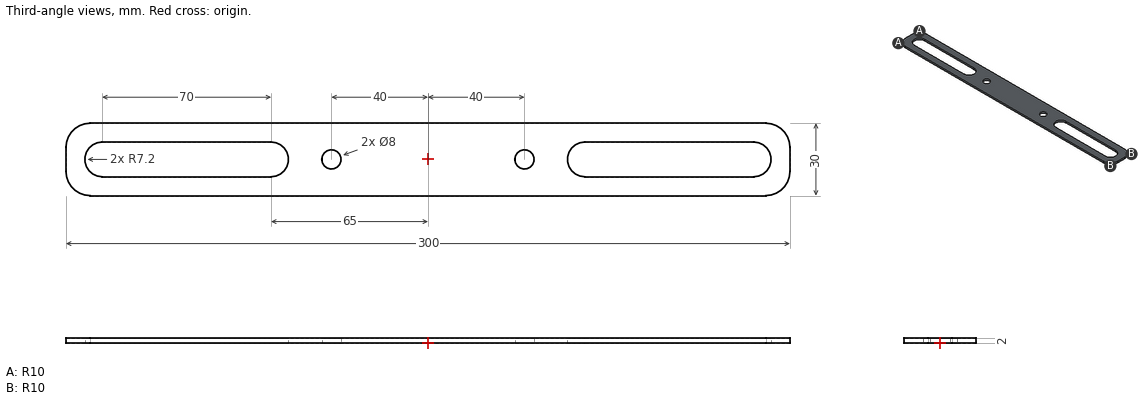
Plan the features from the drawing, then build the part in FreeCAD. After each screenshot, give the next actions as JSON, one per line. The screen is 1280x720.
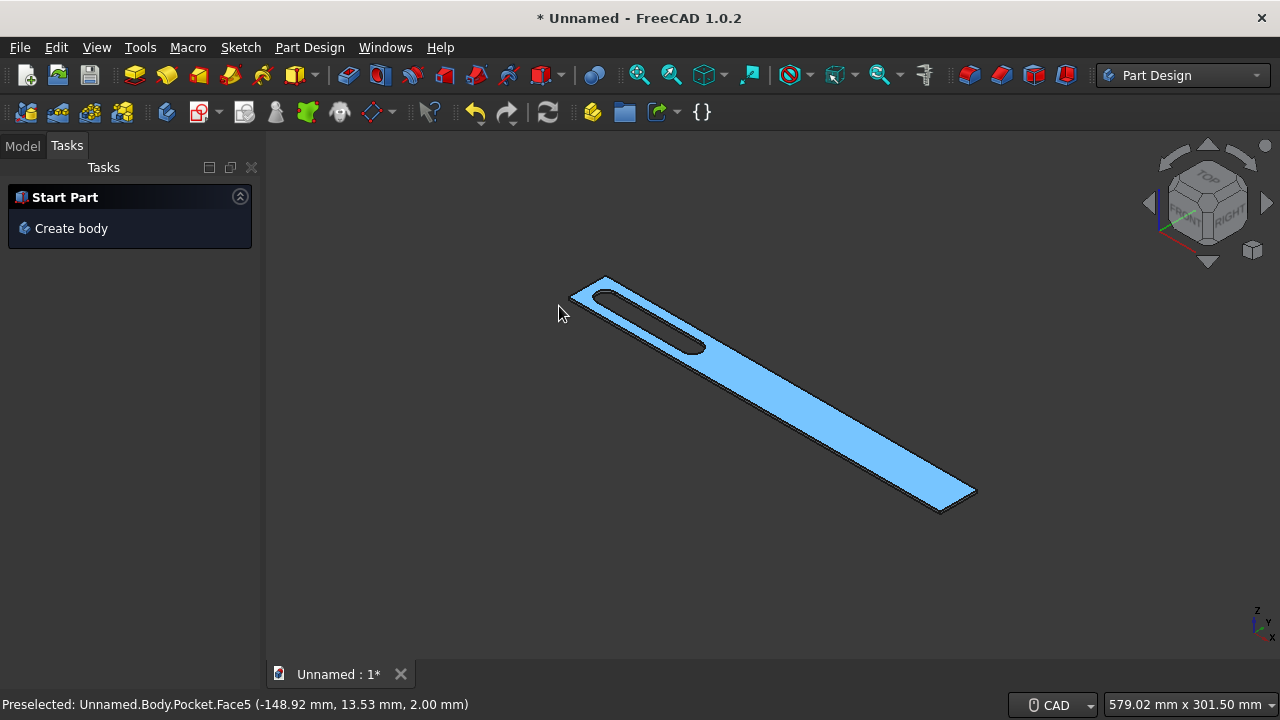
{"action": "scroll", "coordinate": [606, 276], "scroll_direction": "up", "scroll_amount": 13}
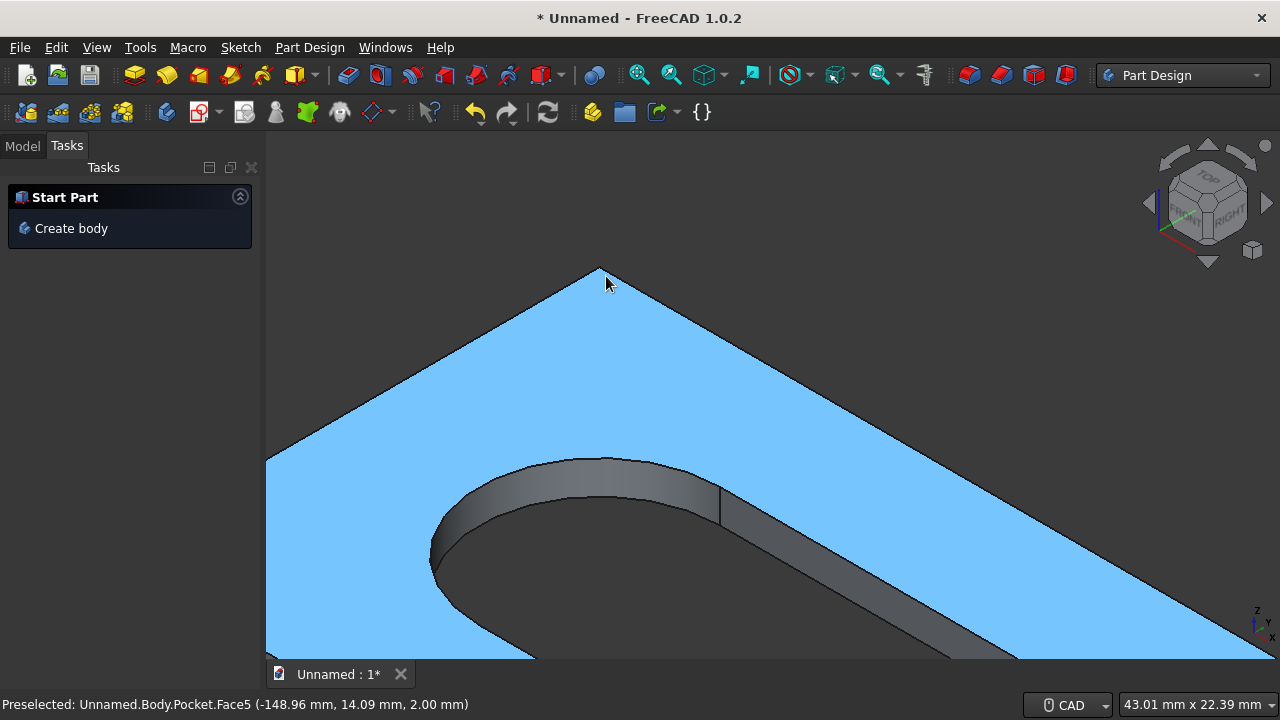
{"action": "left_click", "coordinate": [640, 76]}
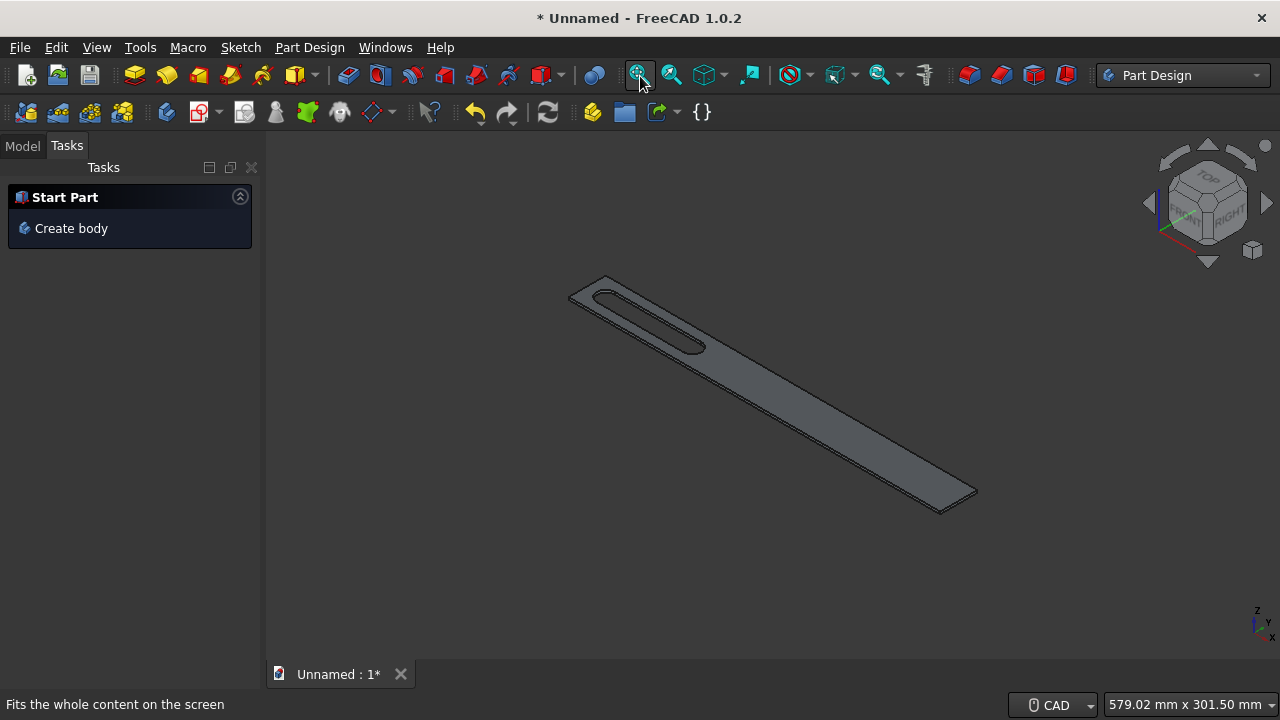
{"action": "key", "text": "2"}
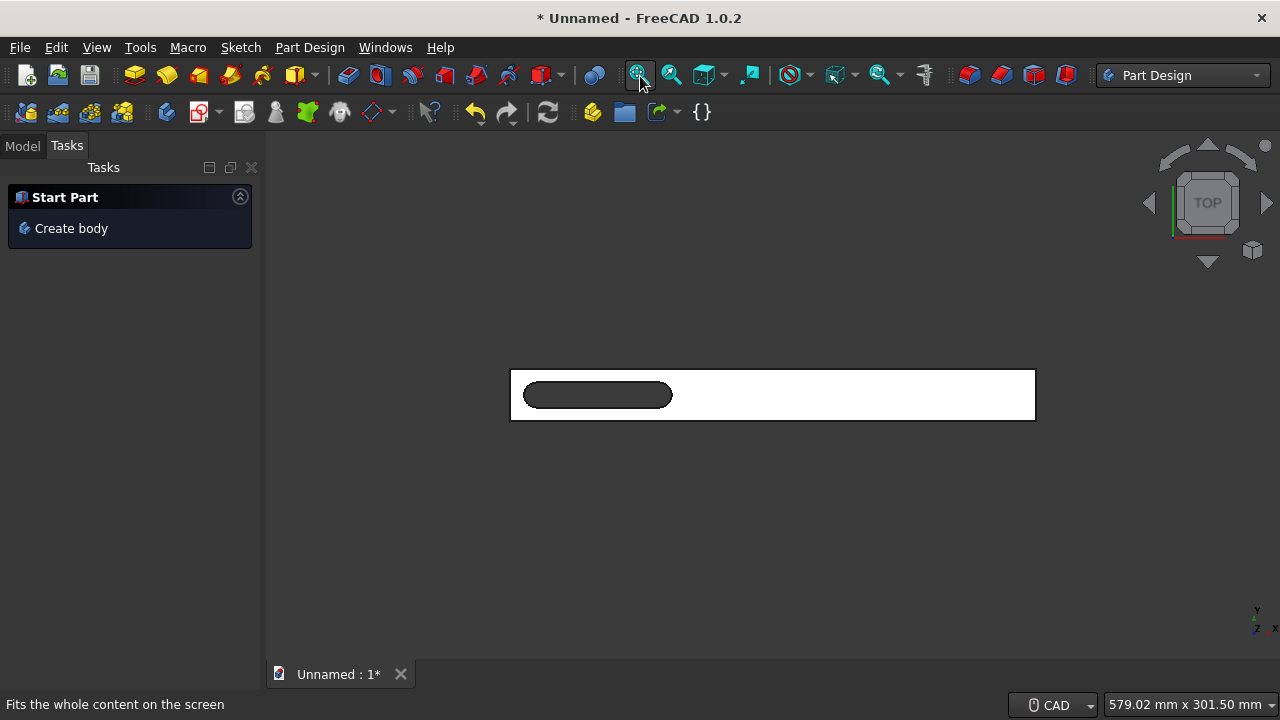
{"action": "scroll", "coordinate": [510, 368], "scroll_direction": "up", "scroll_amount": 13}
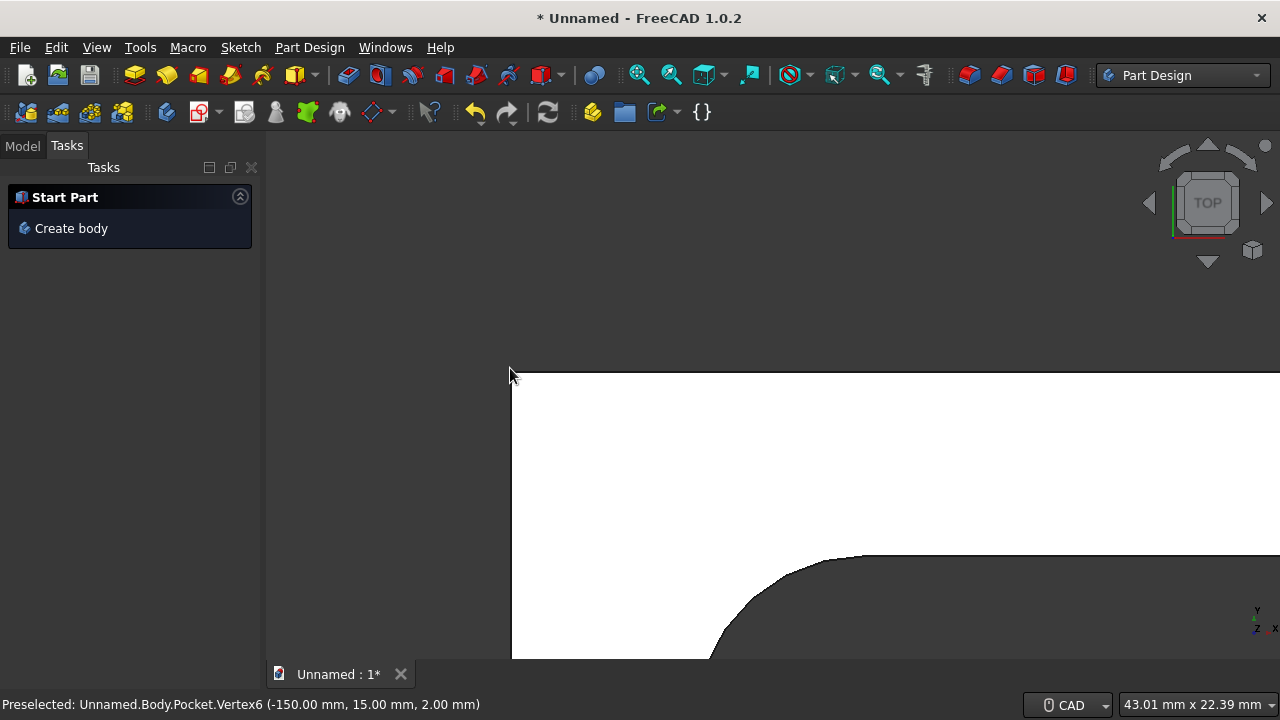
{"action": "key", "text": "v f"}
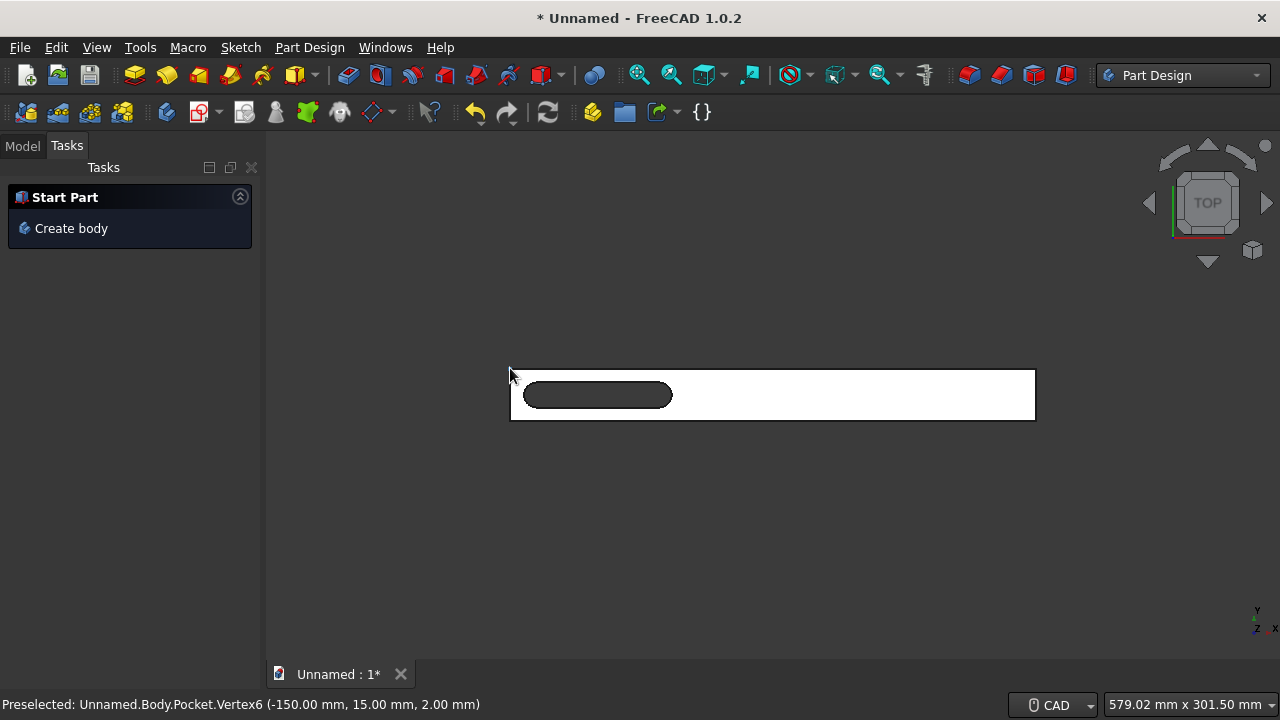
{"action": "key", "text": "1"}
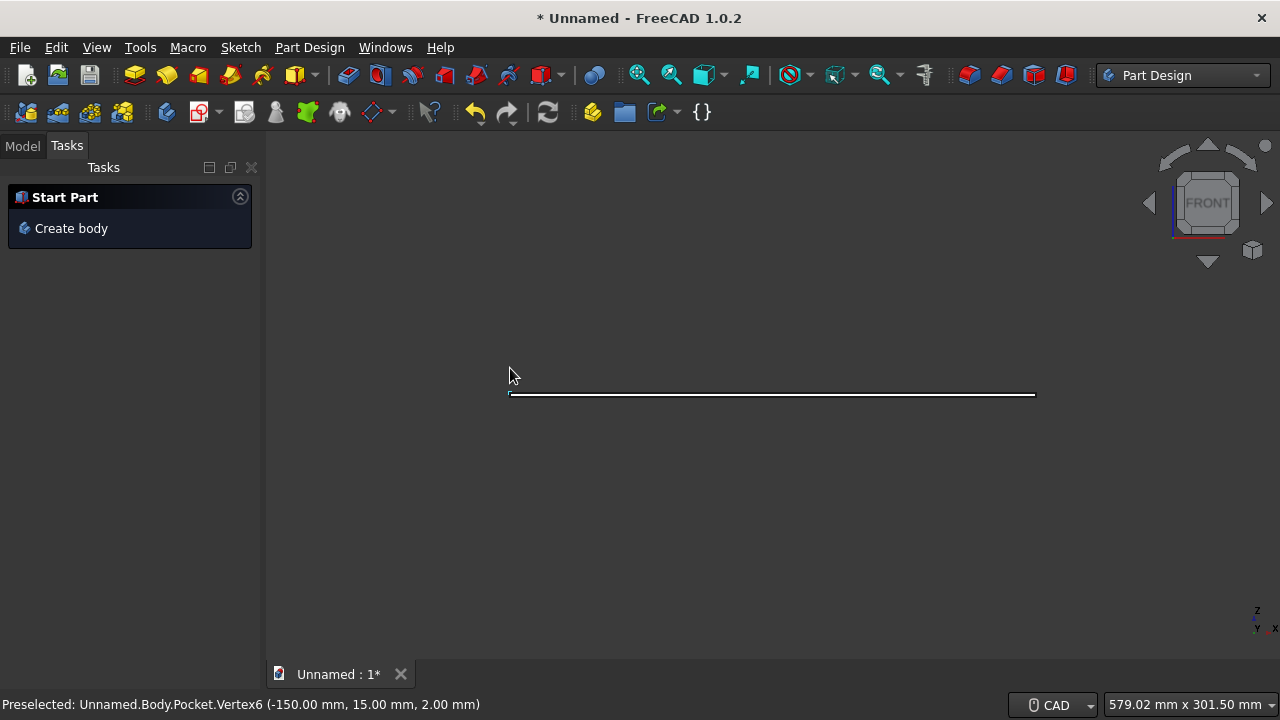
{"action": "scroll", "coordinate": [510, 394], "scroll_direction": "up", "scroll_amount": 13}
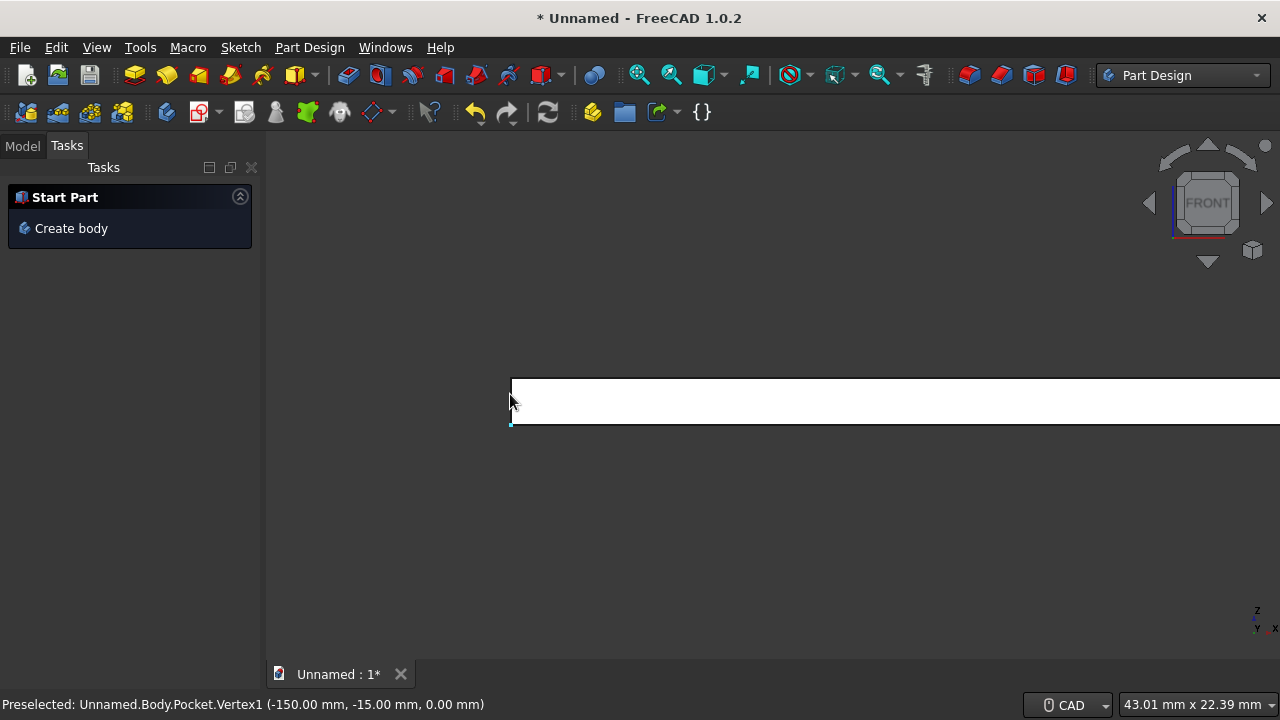
{"action": "left_click", "coordinate": [511, 400]}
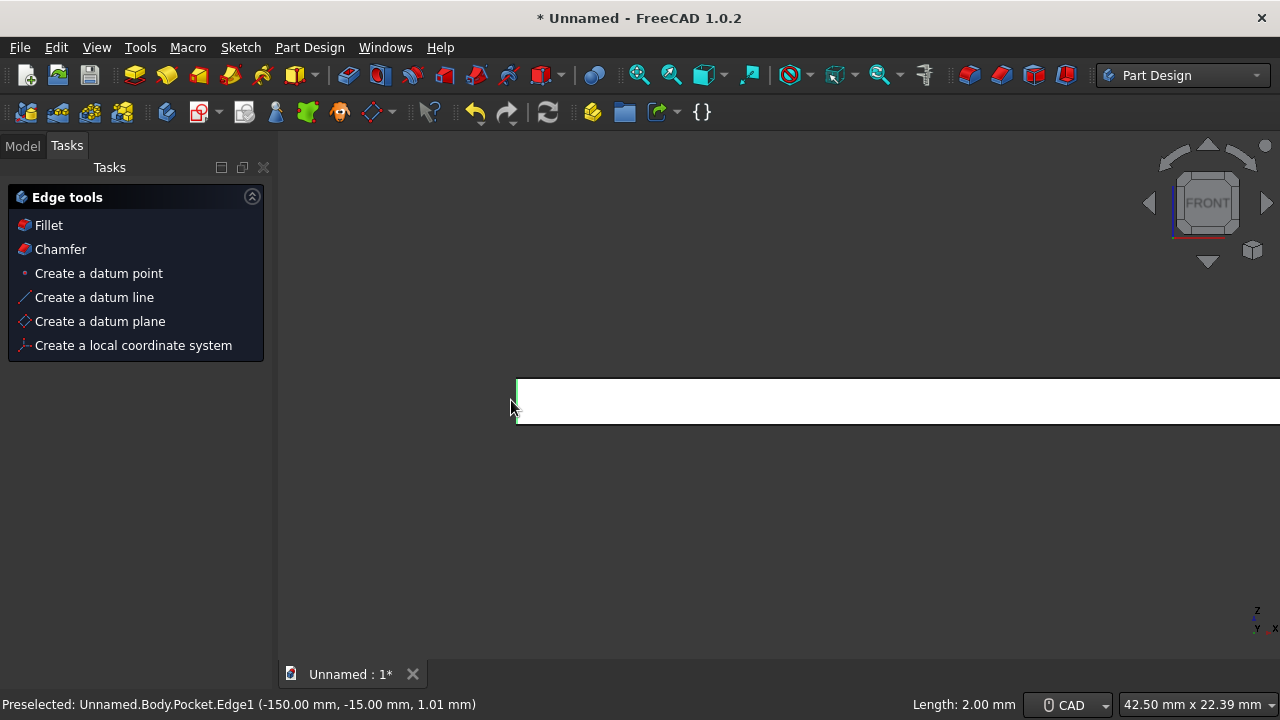
{"action": "left_click", "coordinate": [640, 76]}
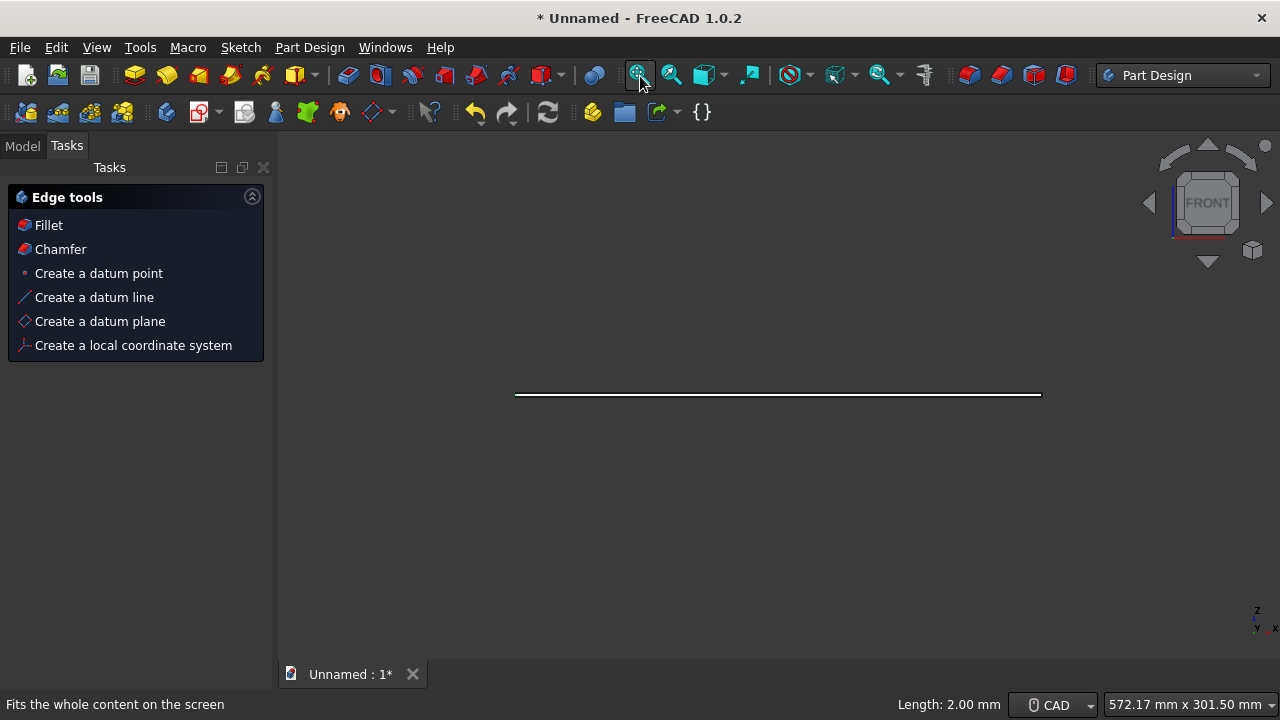
{"action": "key", "text": "3"}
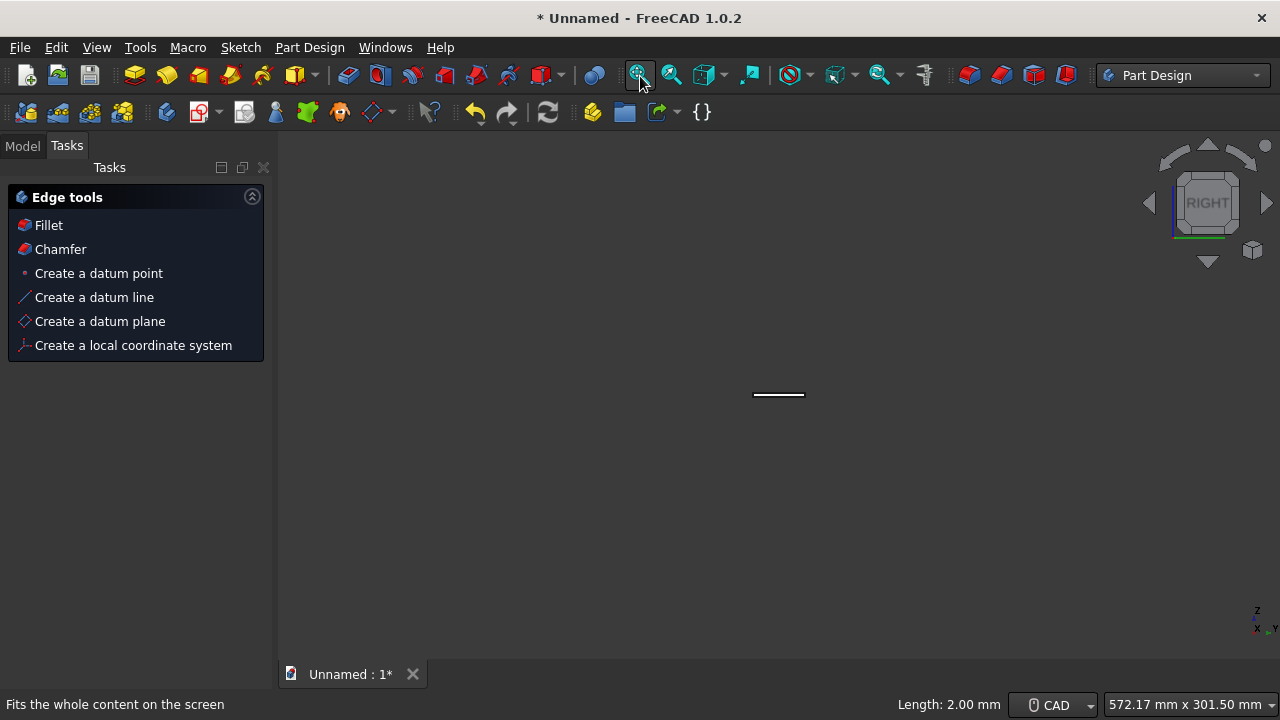
{"action": "key", "text": "v f"}